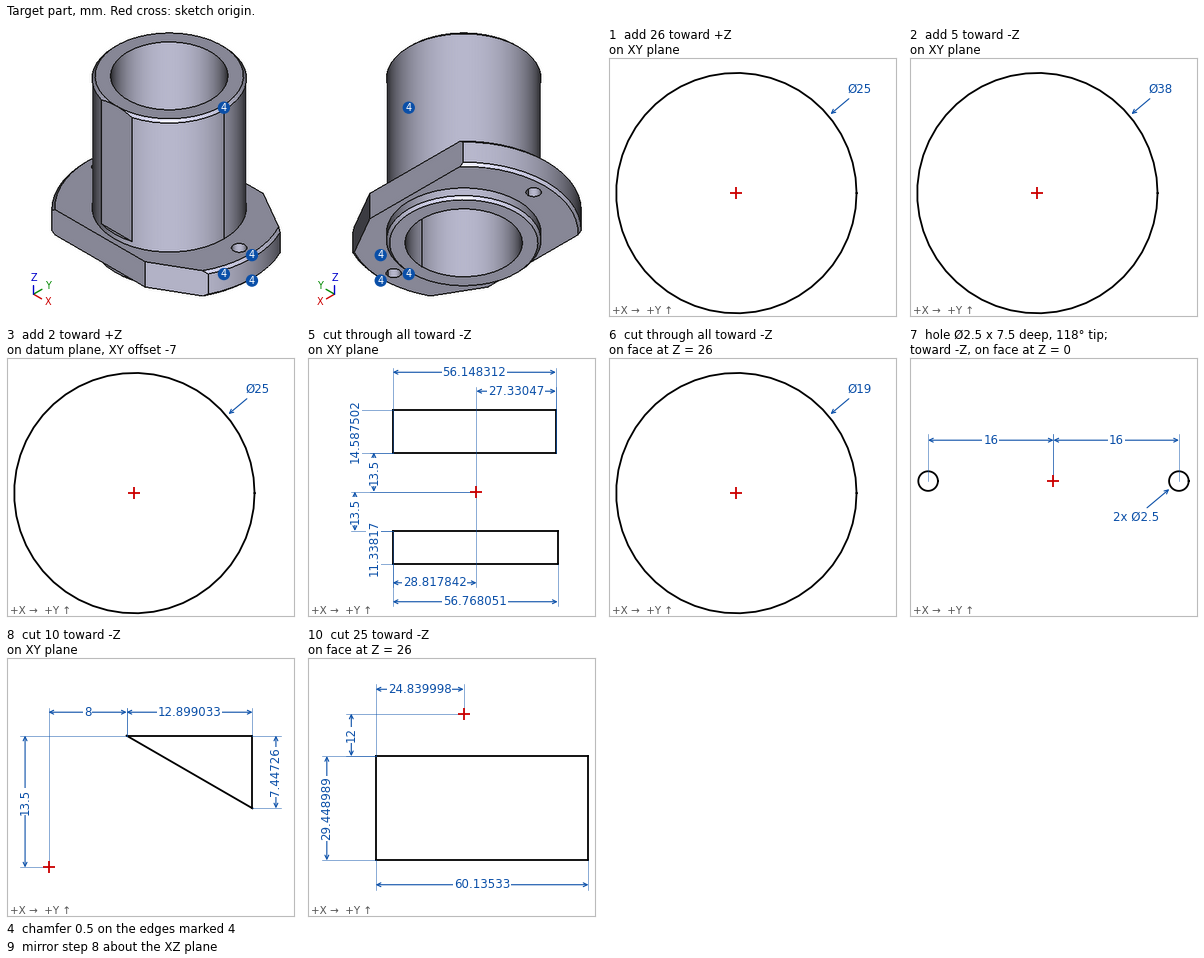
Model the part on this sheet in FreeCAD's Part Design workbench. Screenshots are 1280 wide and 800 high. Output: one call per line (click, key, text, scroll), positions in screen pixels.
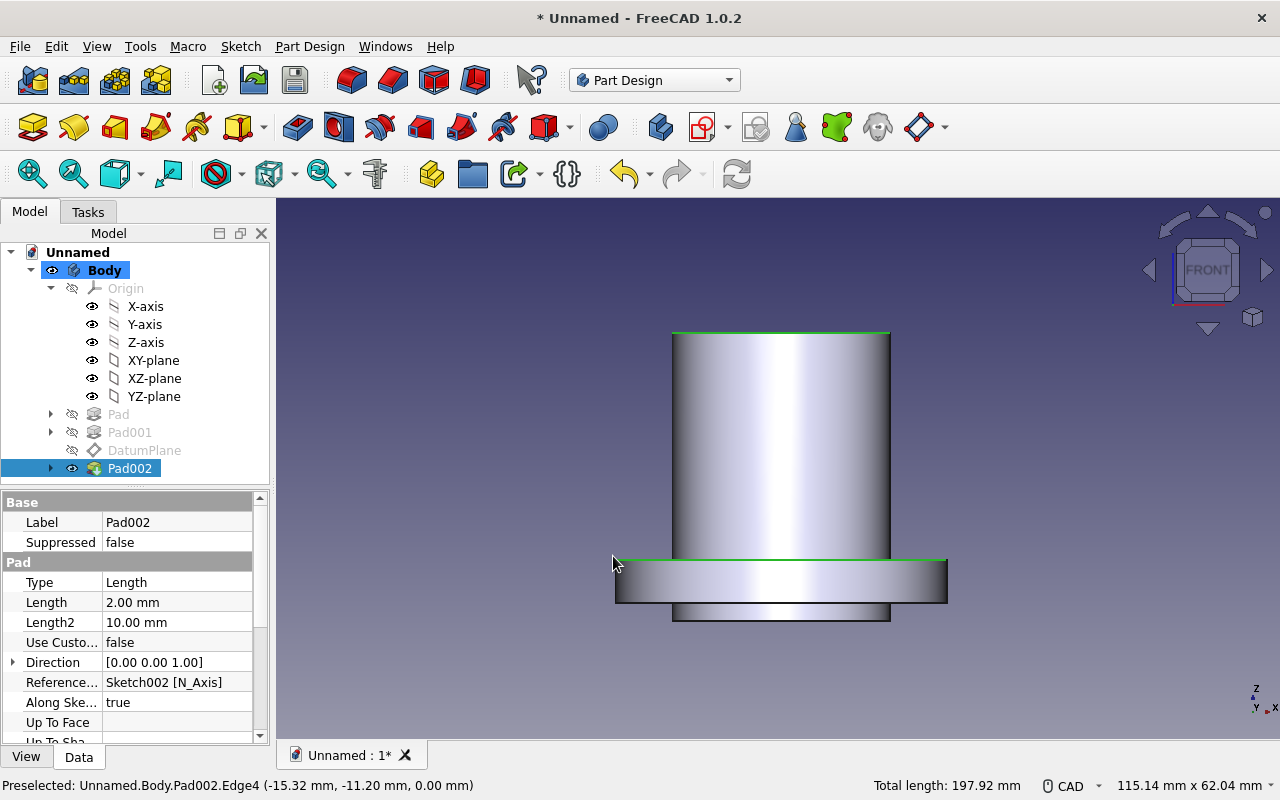
click(693, 620, ctrl)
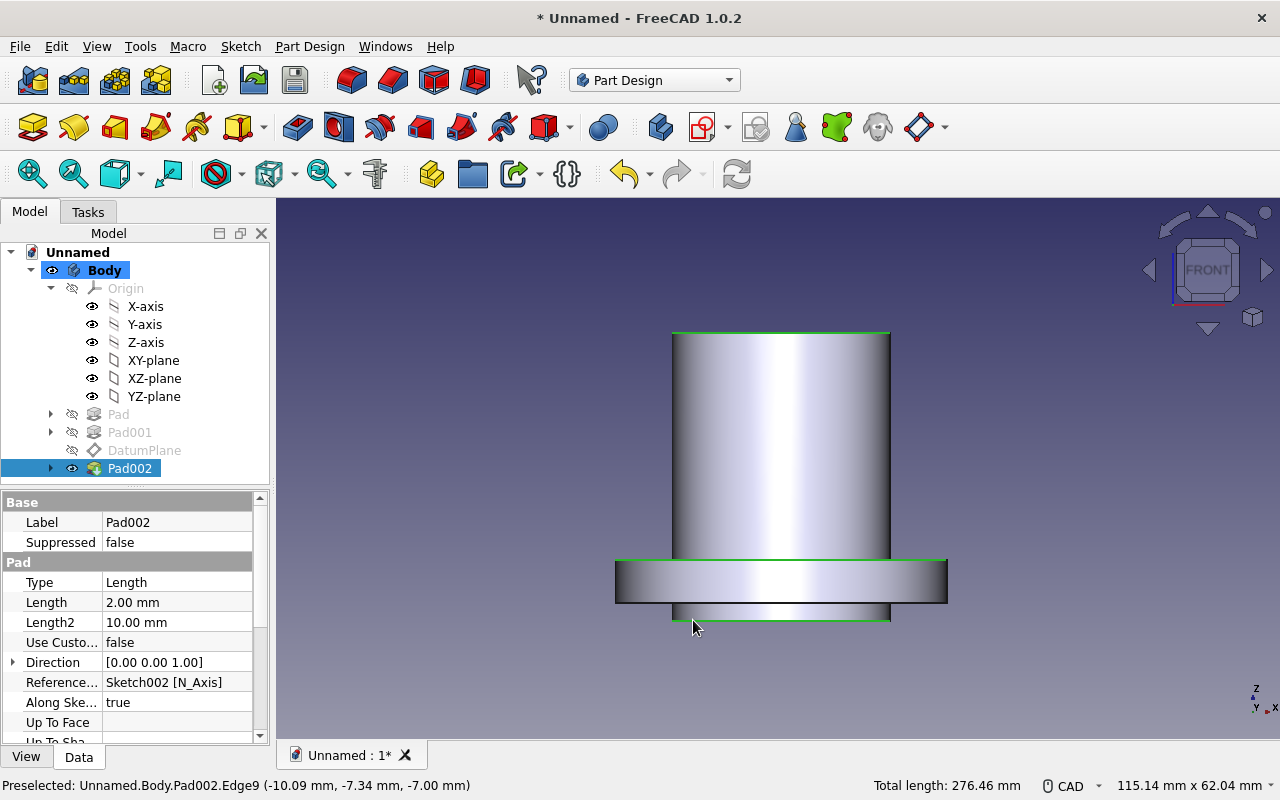
click(647, 602, ctrl)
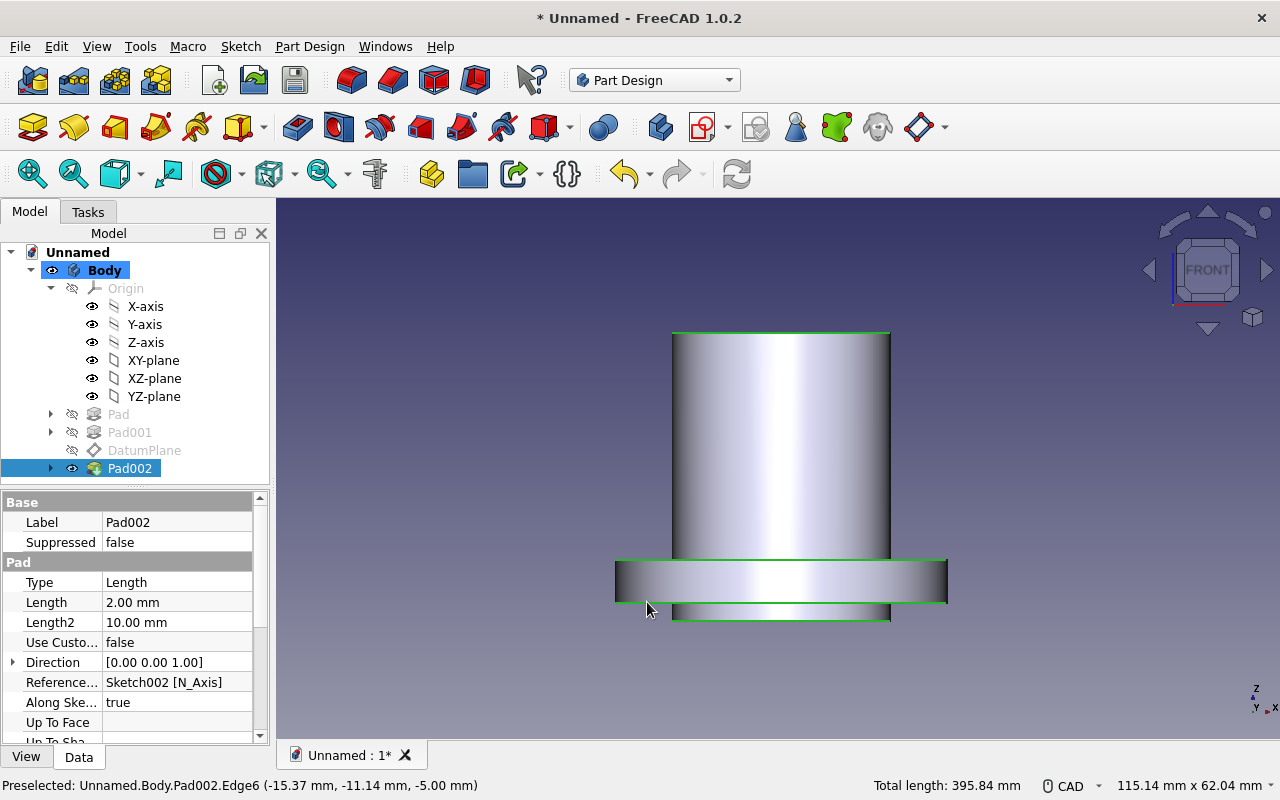
click(393, 80)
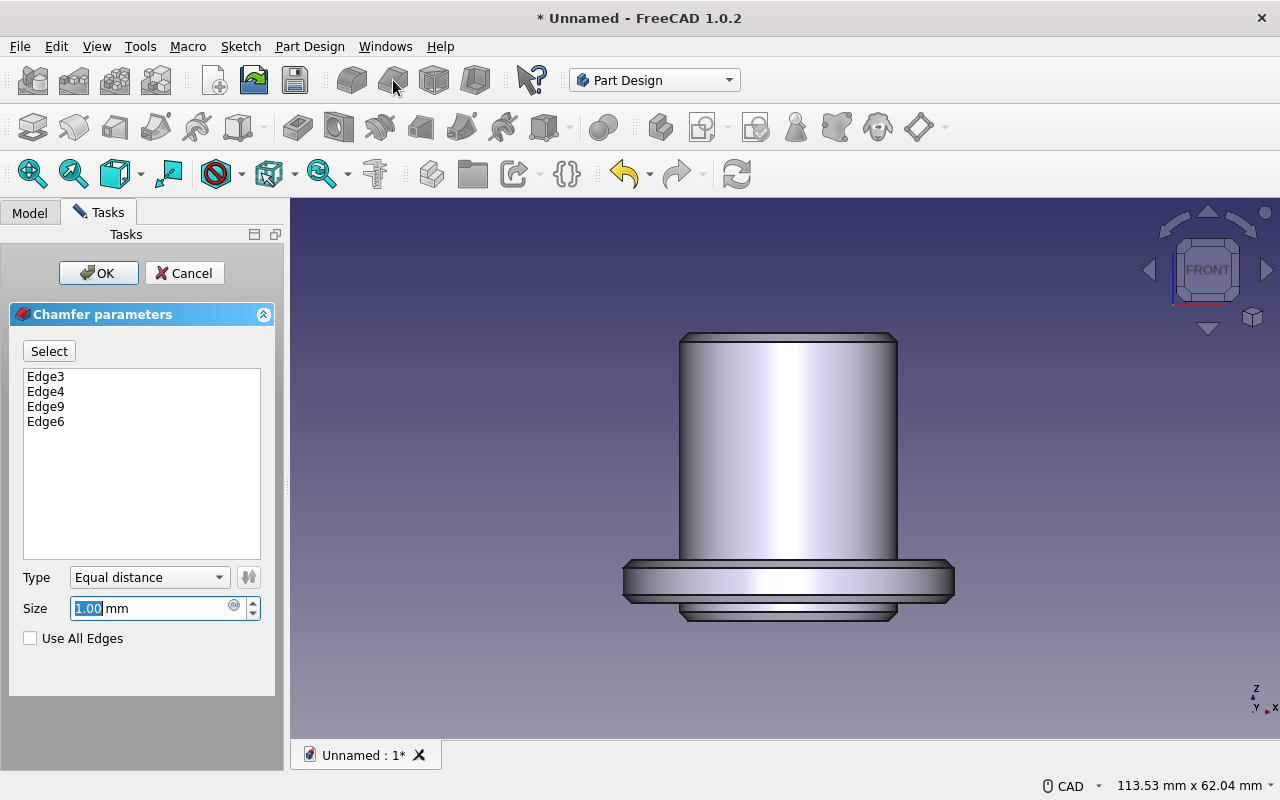
text(0.5)
key(Tab)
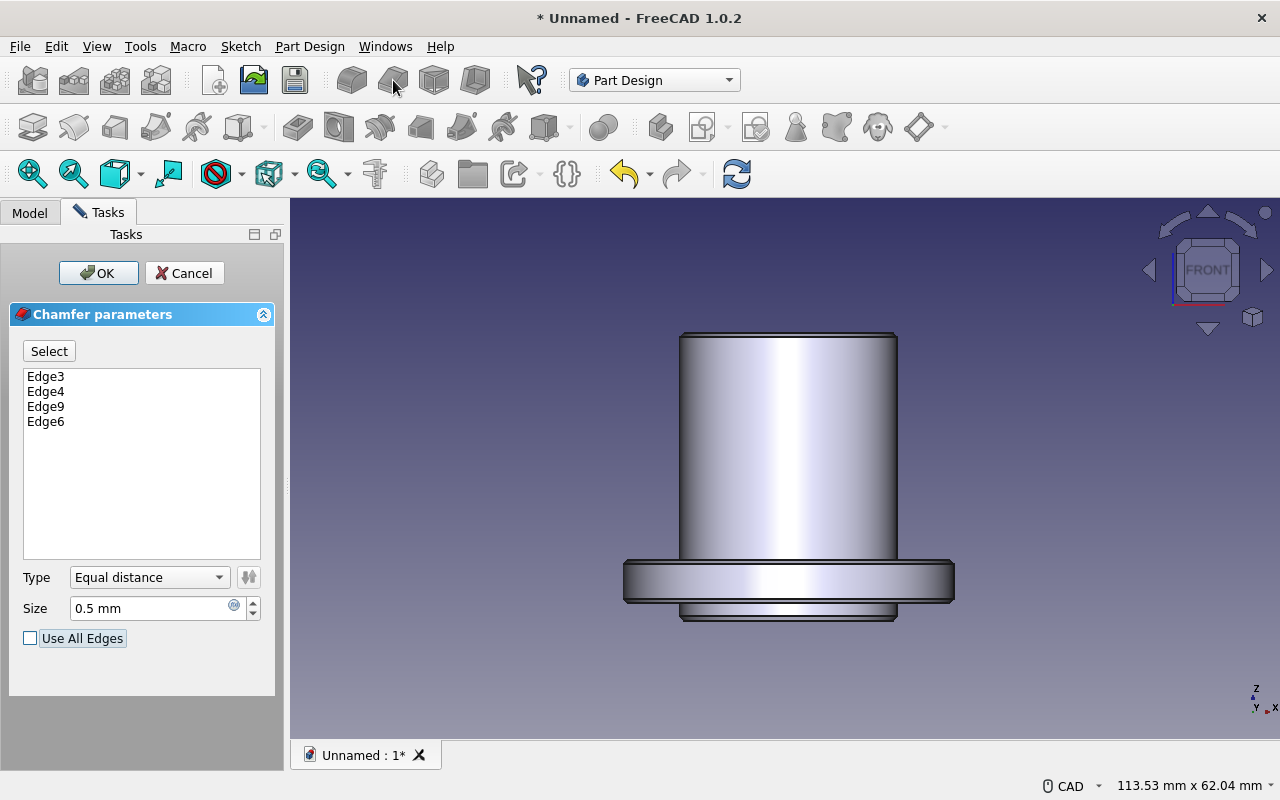
click(99, 273)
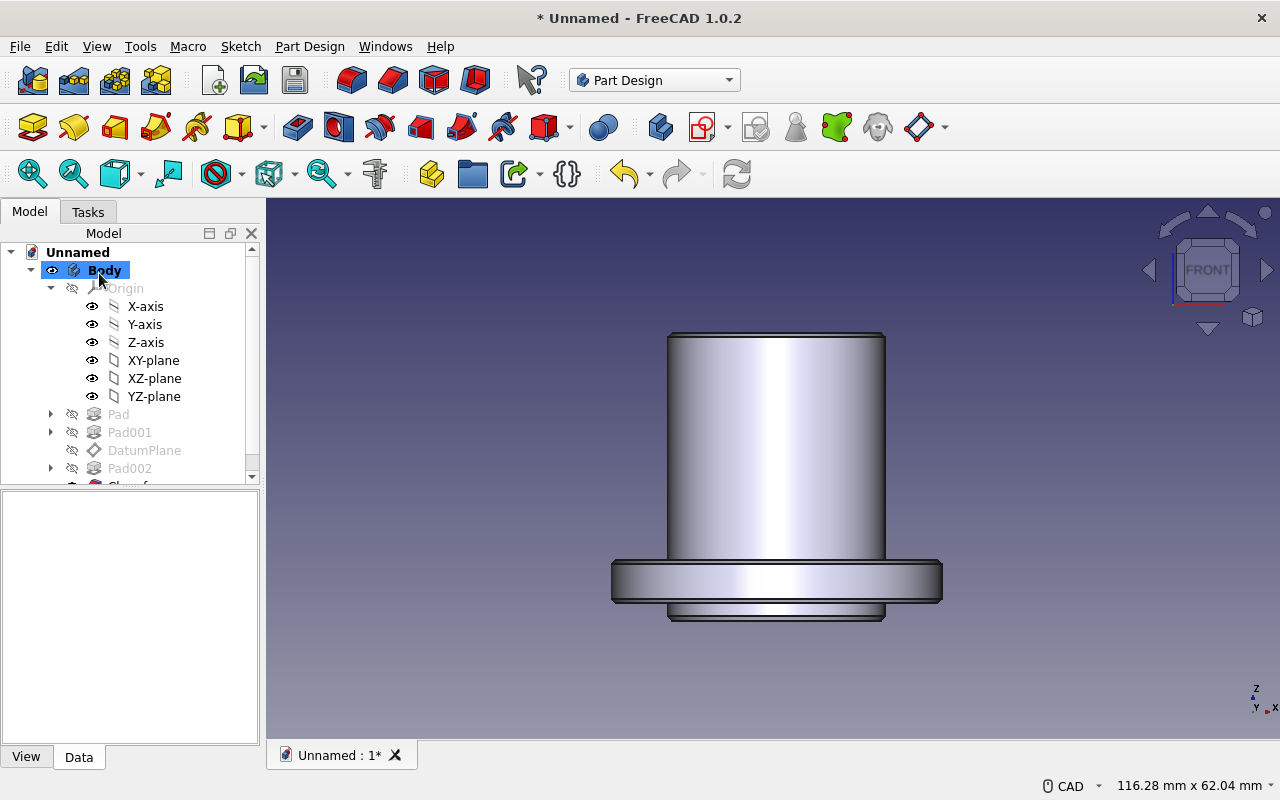
click(702, 128)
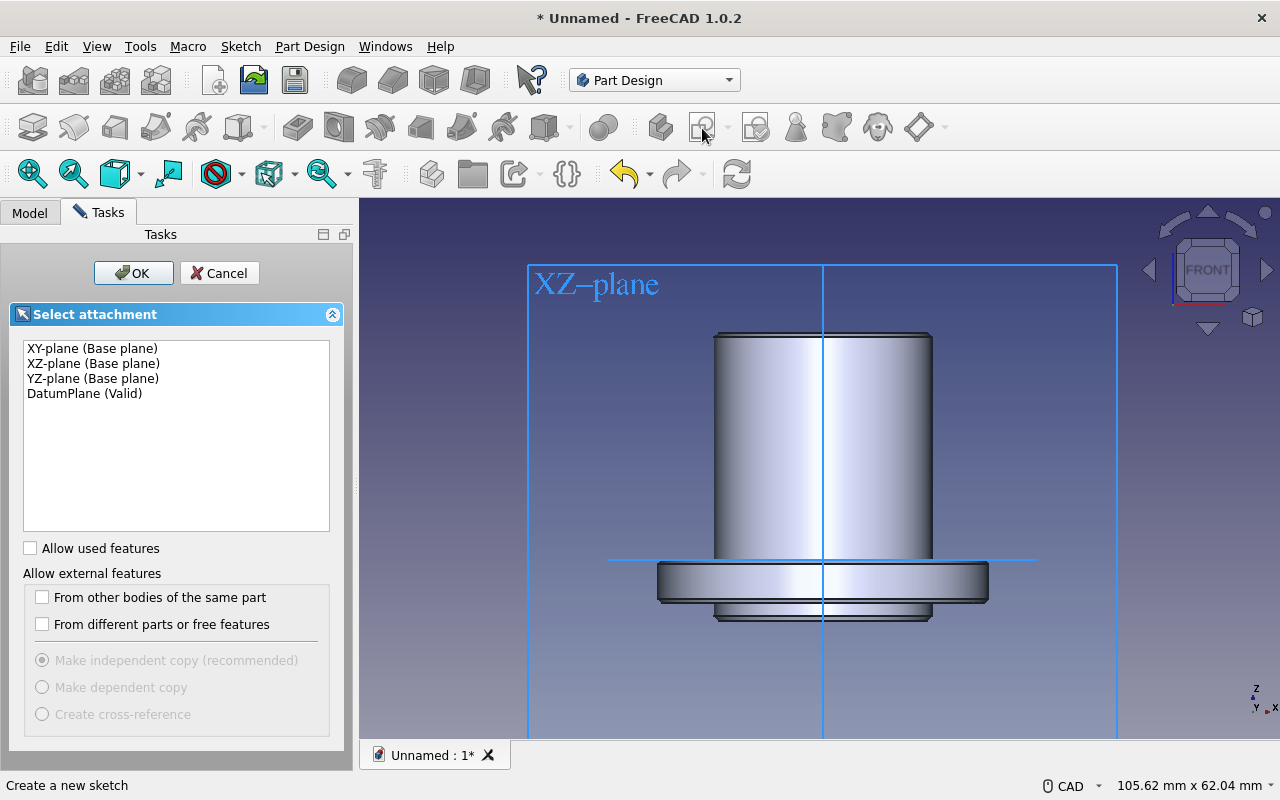
click(84, 348)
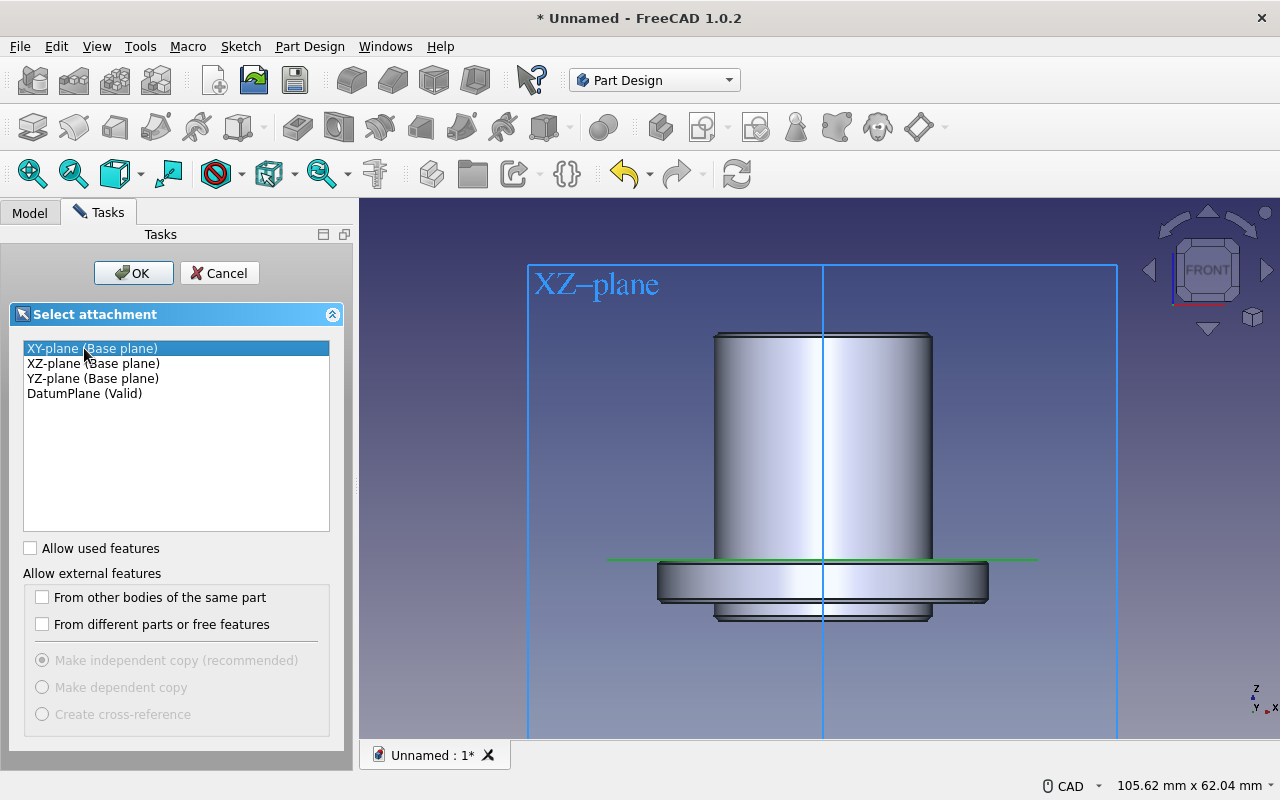
click(134, 273)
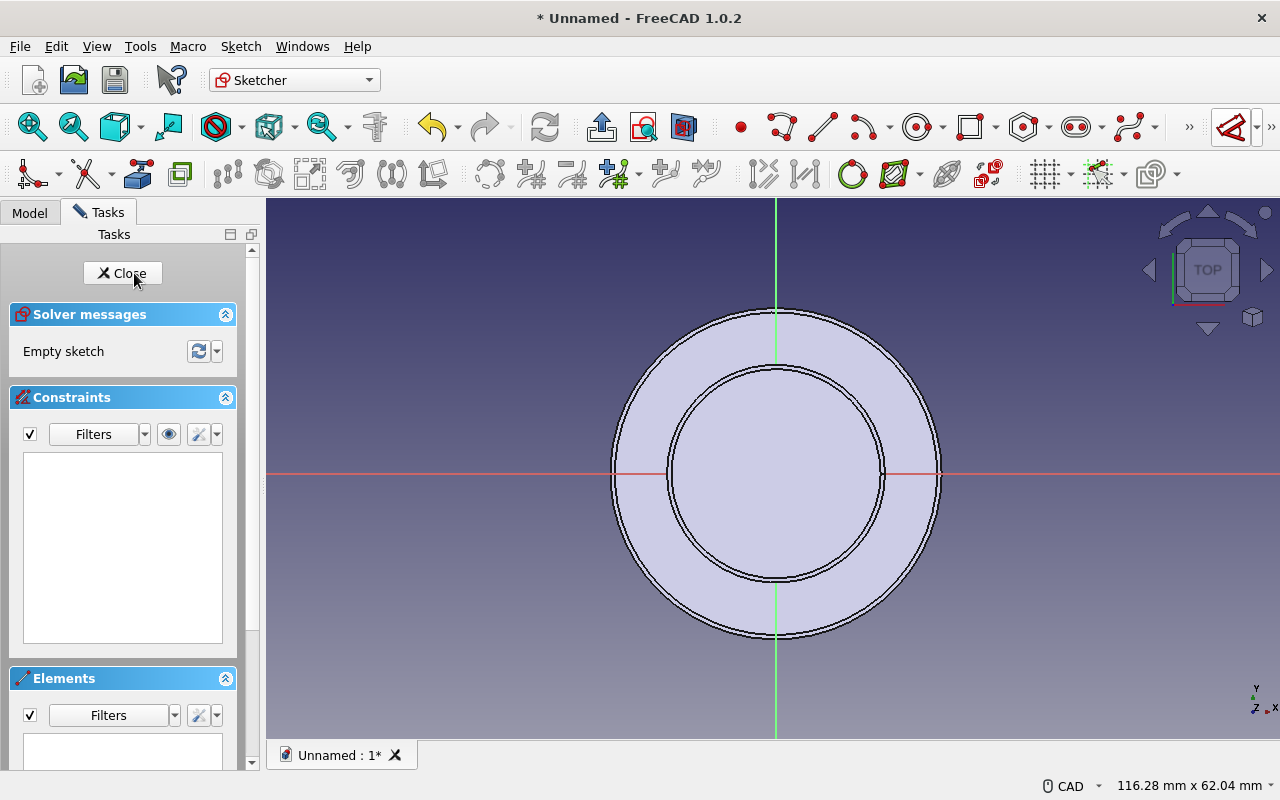
key(q)
key(s)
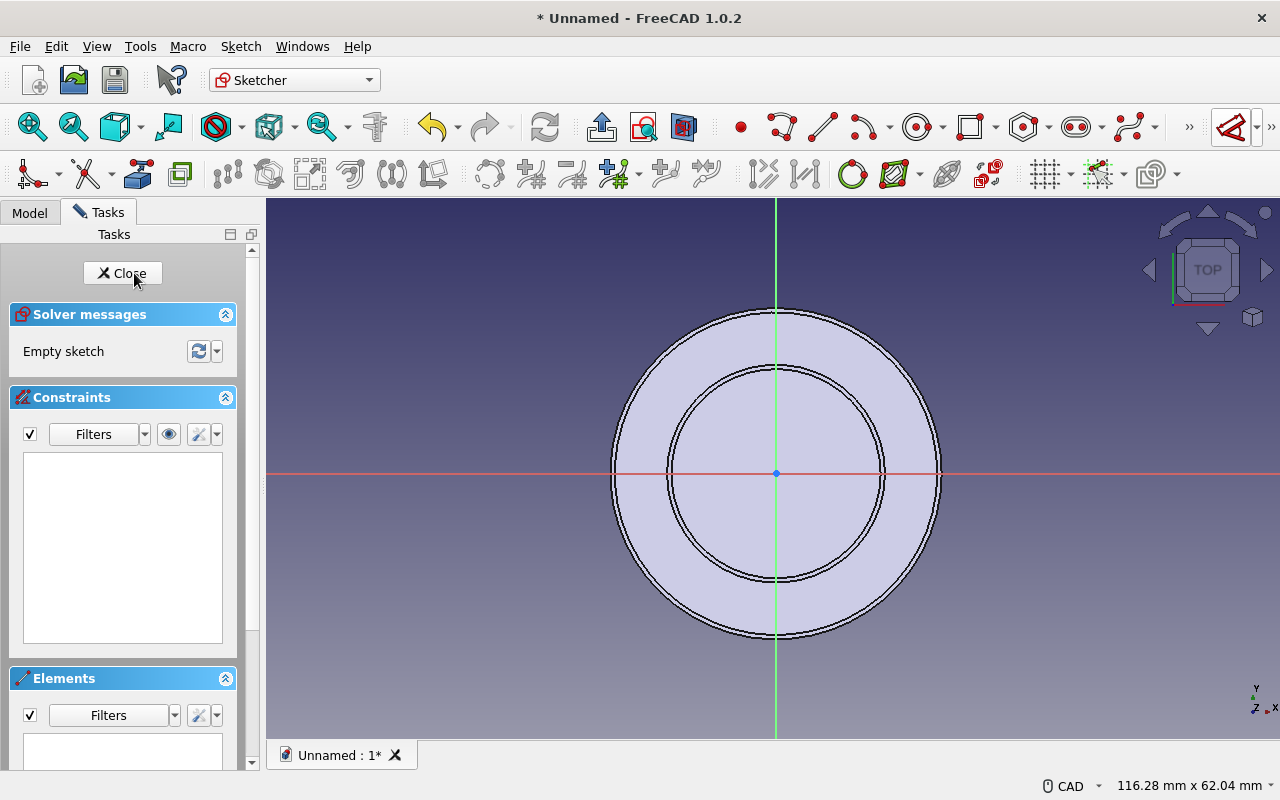
scroll(399, 509, down, 1)